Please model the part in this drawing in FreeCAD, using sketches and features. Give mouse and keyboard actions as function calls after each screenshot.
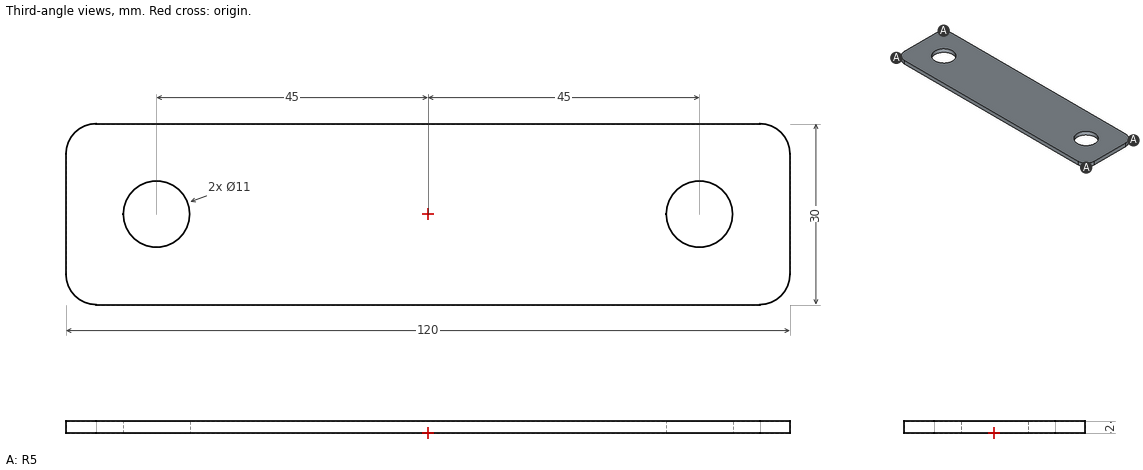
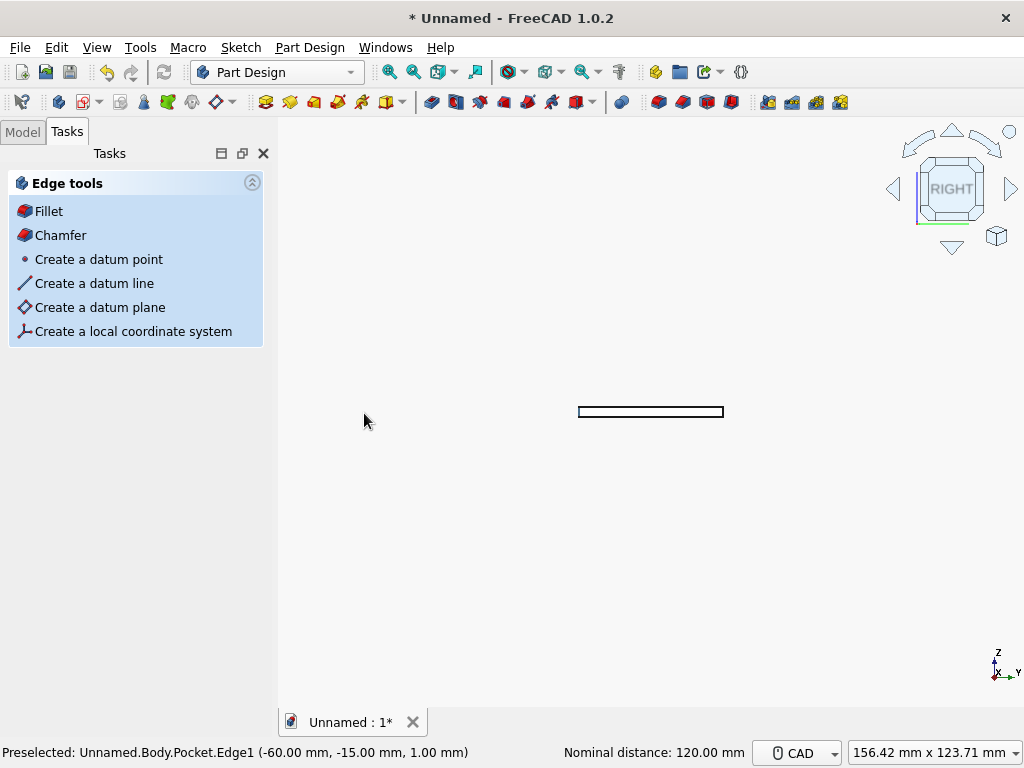
key(v)
key(f)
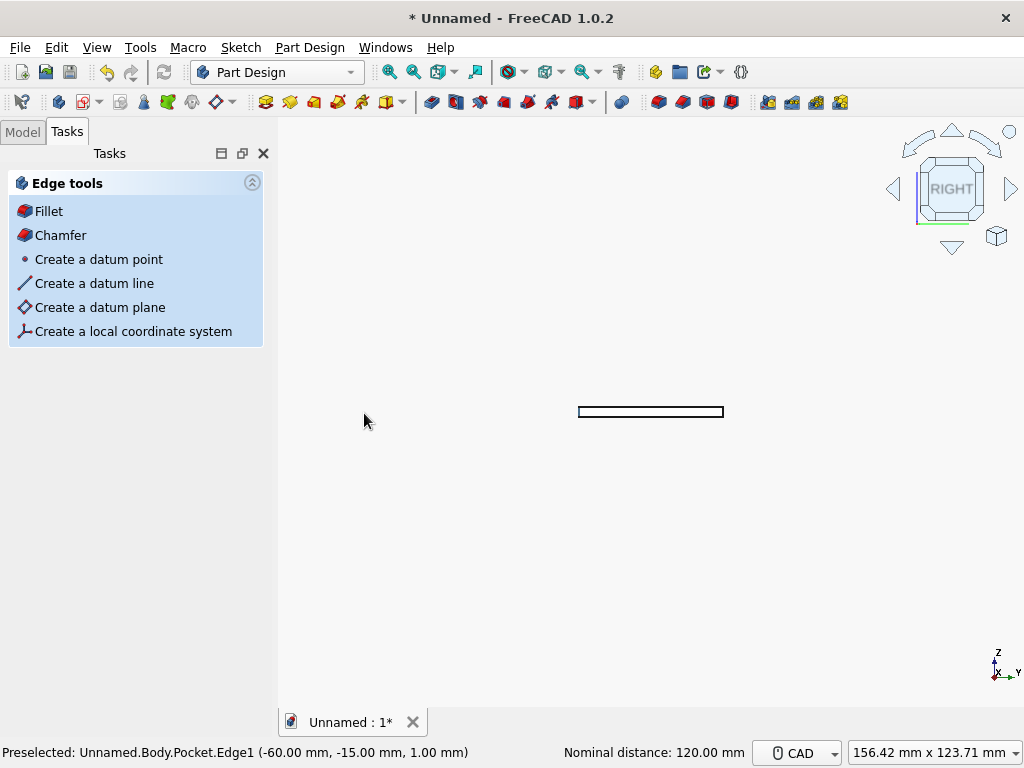
scroll(723, 411, up, 8)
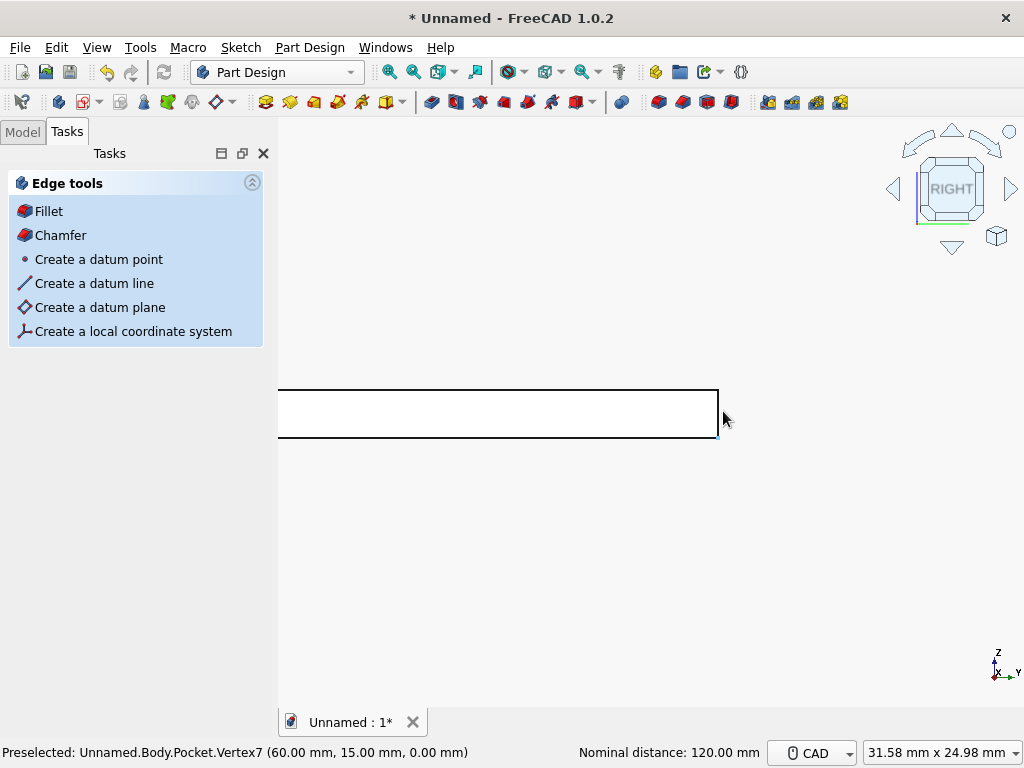
click(718, 413, ctrl)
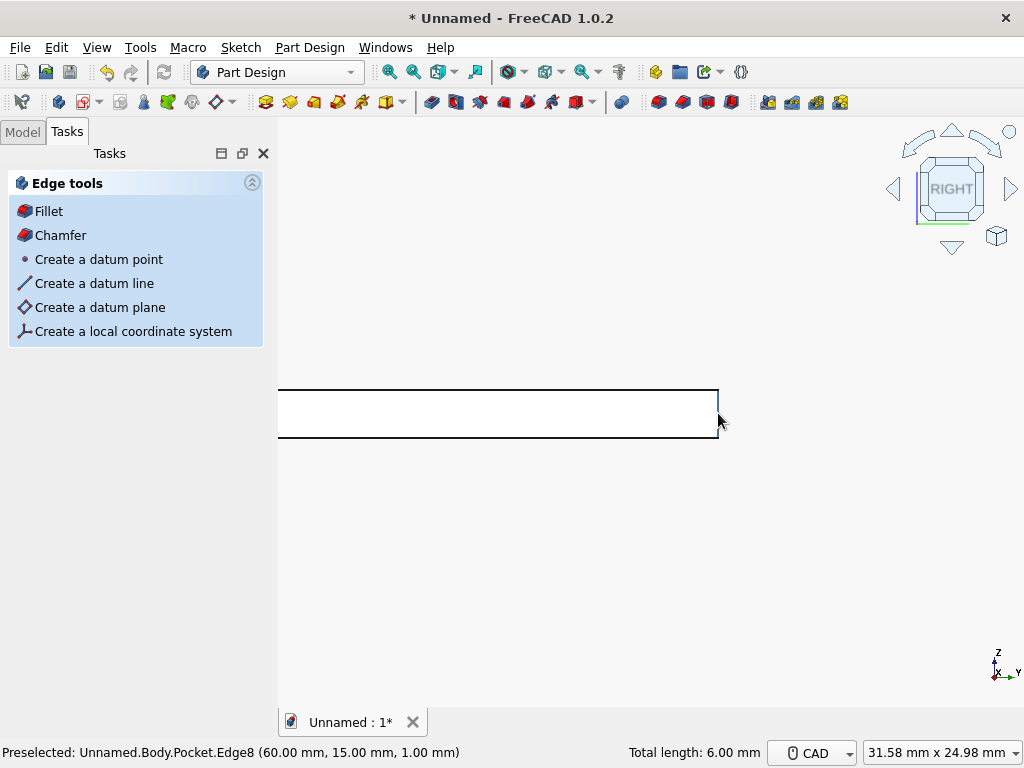
key(v)
key(f)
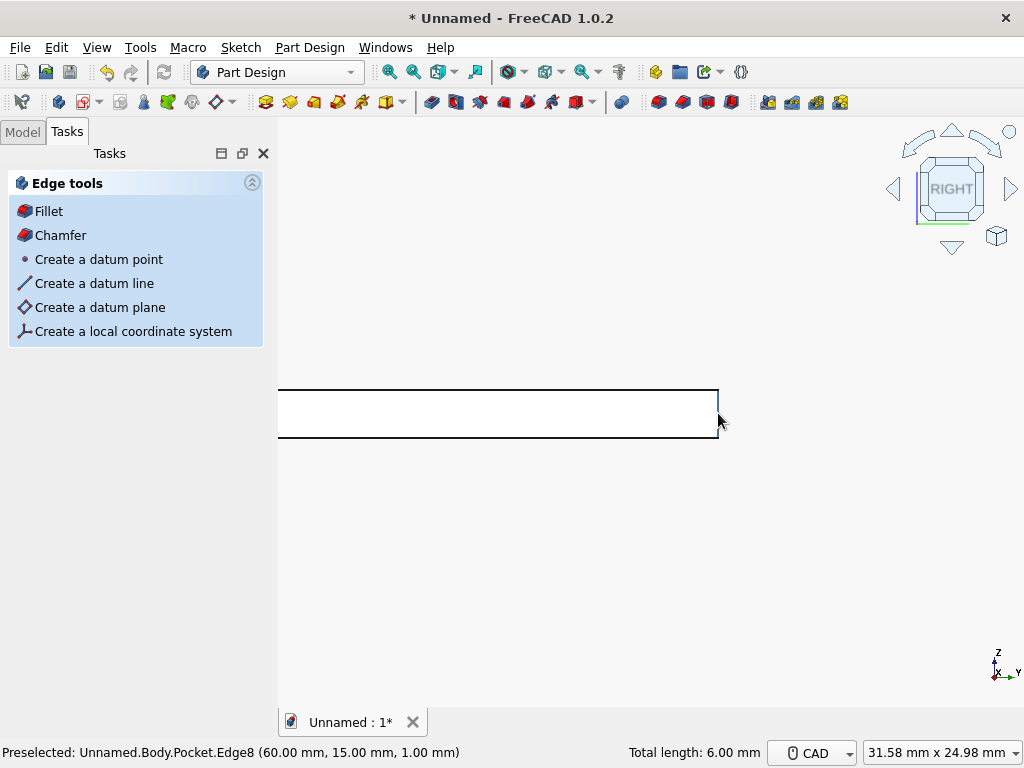
key(5)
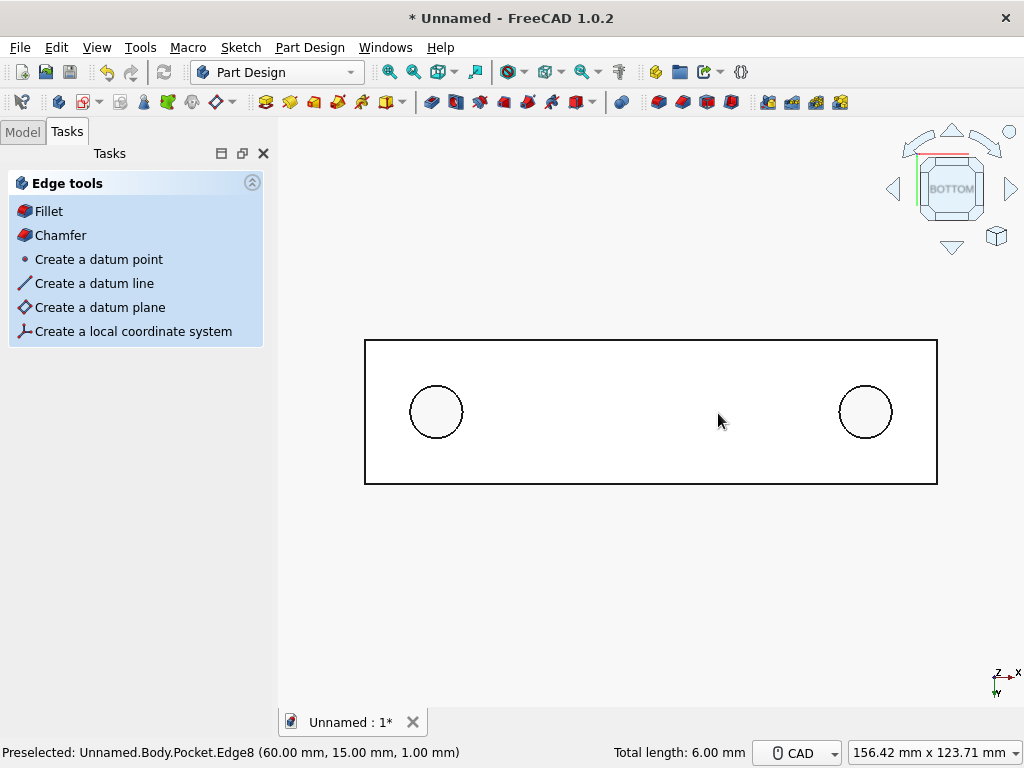
scroll(365, 483, up, 8)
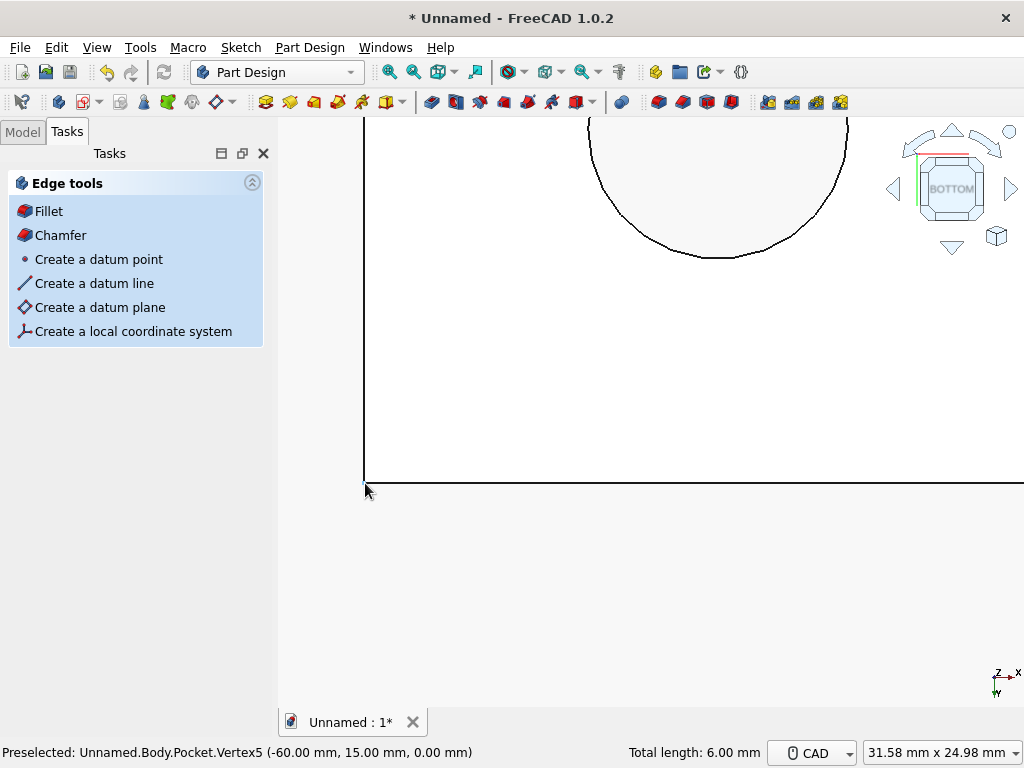
key(v)
key(f)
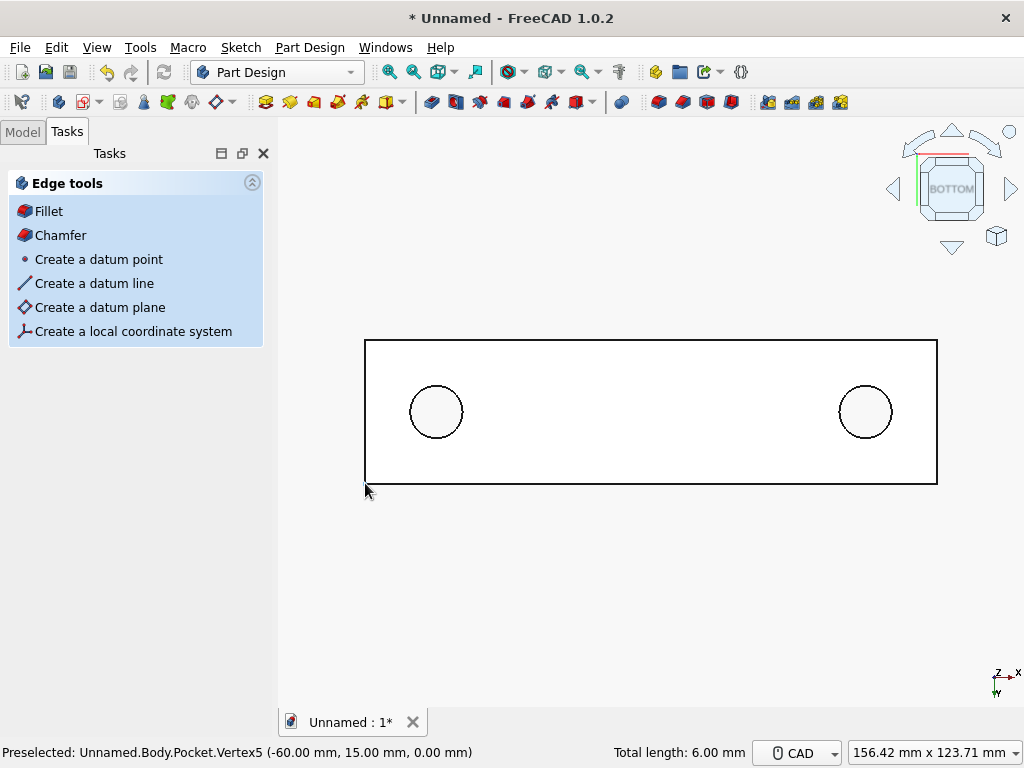
key(4)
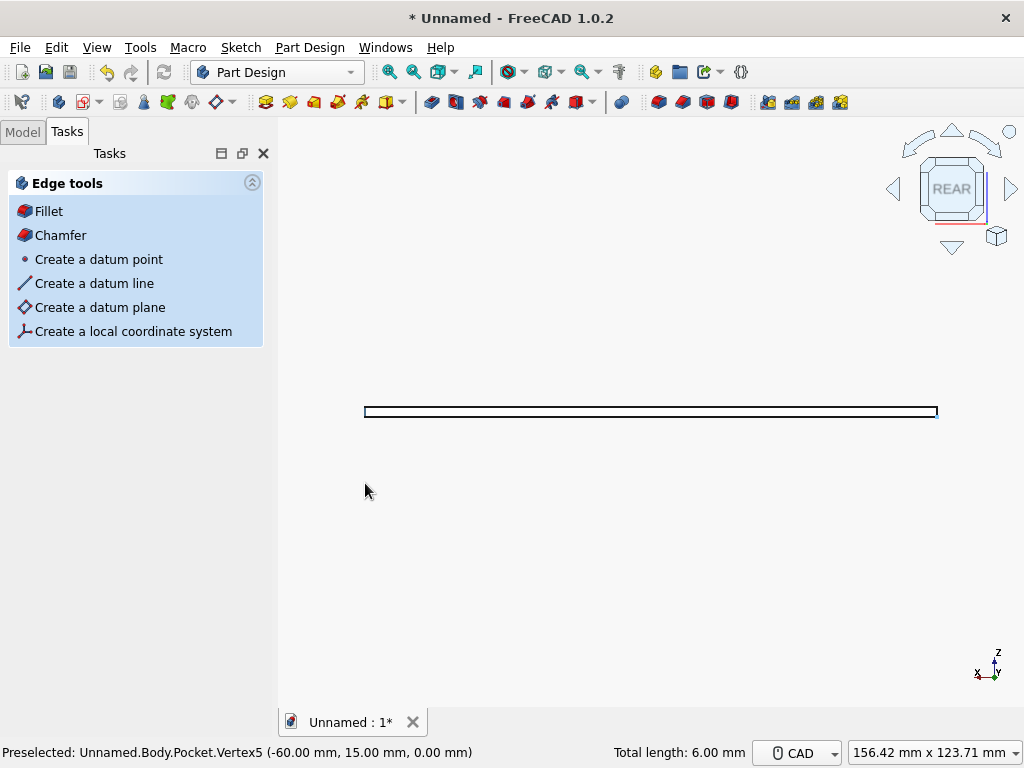
key(6)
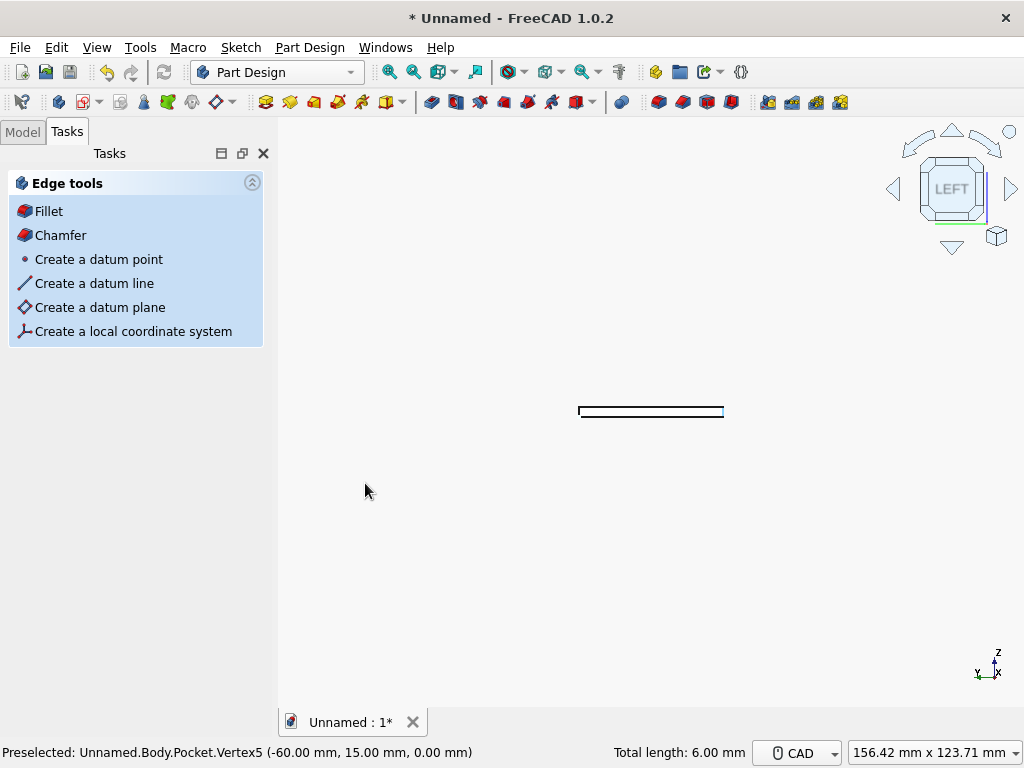
click(390, 72)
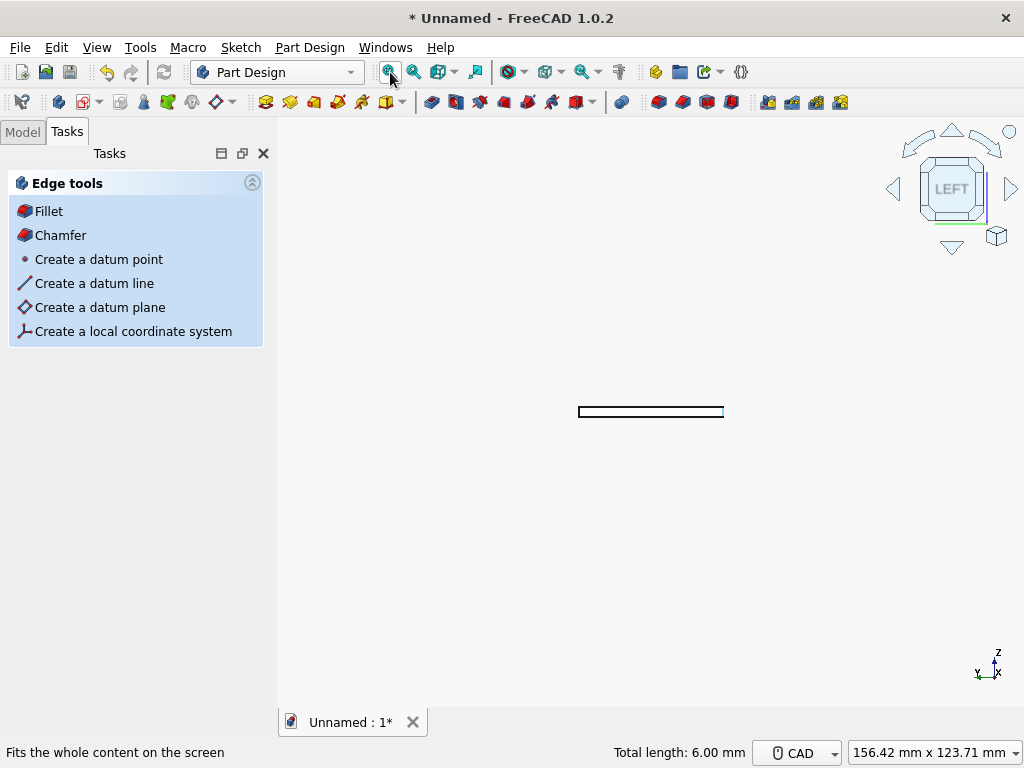
scroll(579, 411, up, 8)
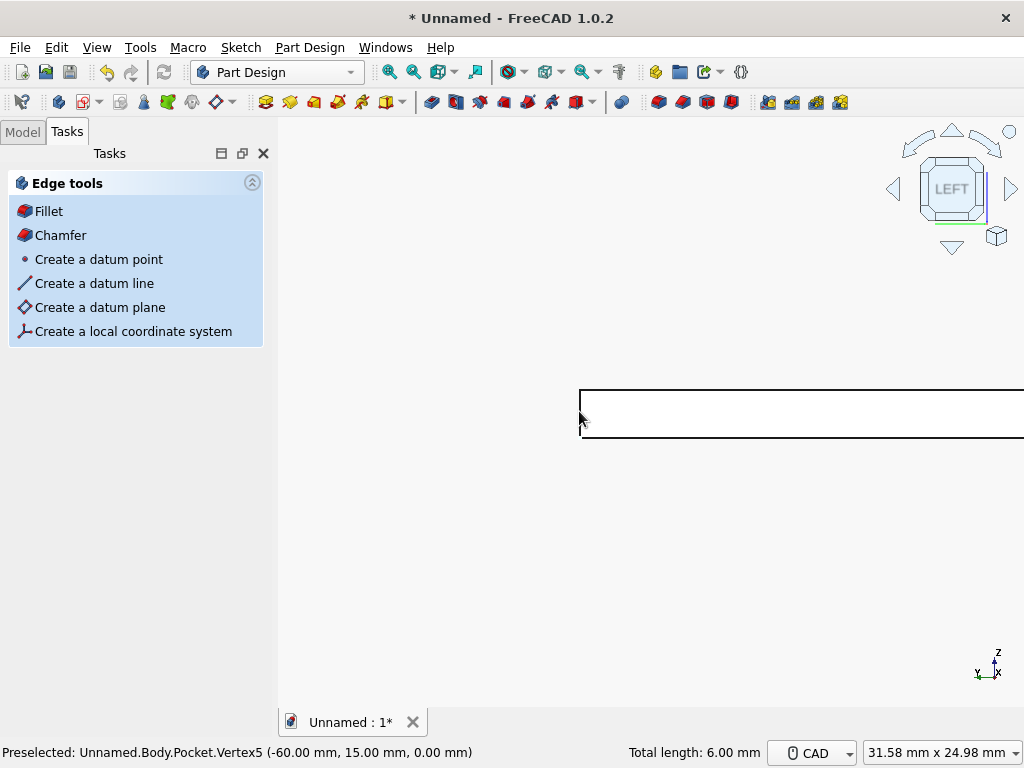
click(580, 413, ctrl)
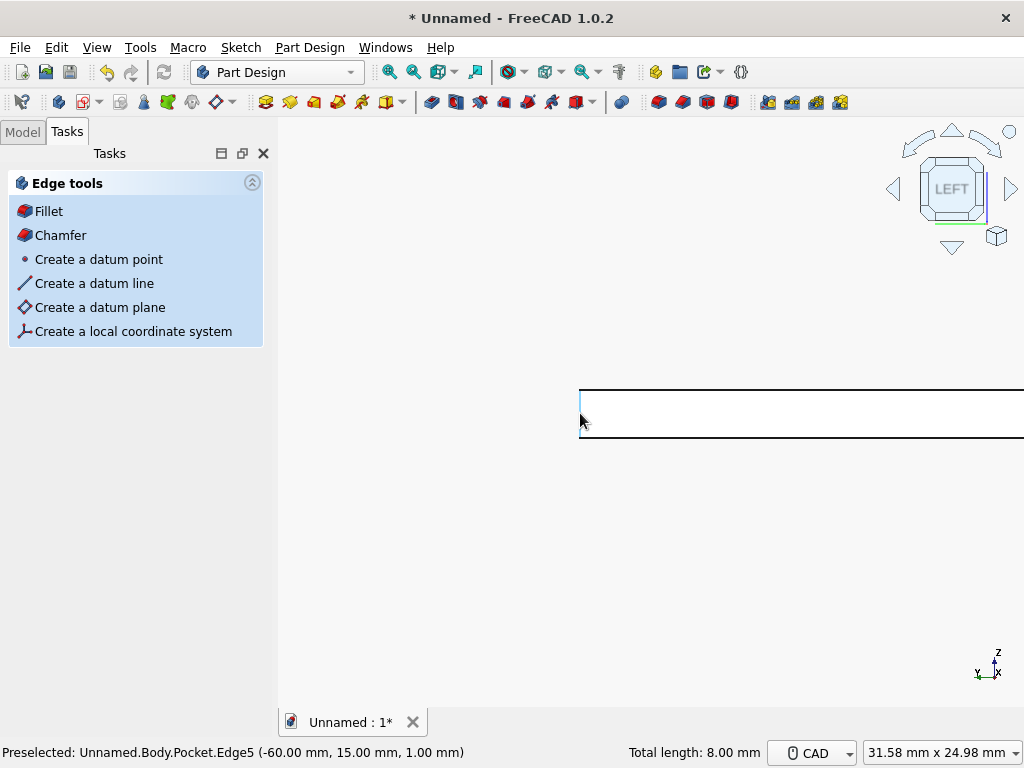
click(660, 102)